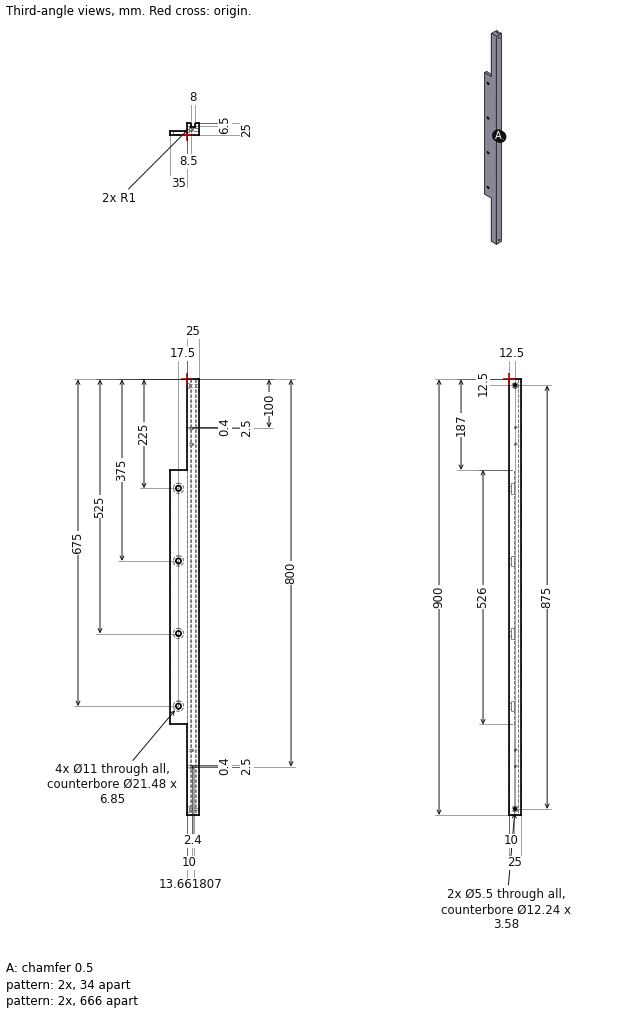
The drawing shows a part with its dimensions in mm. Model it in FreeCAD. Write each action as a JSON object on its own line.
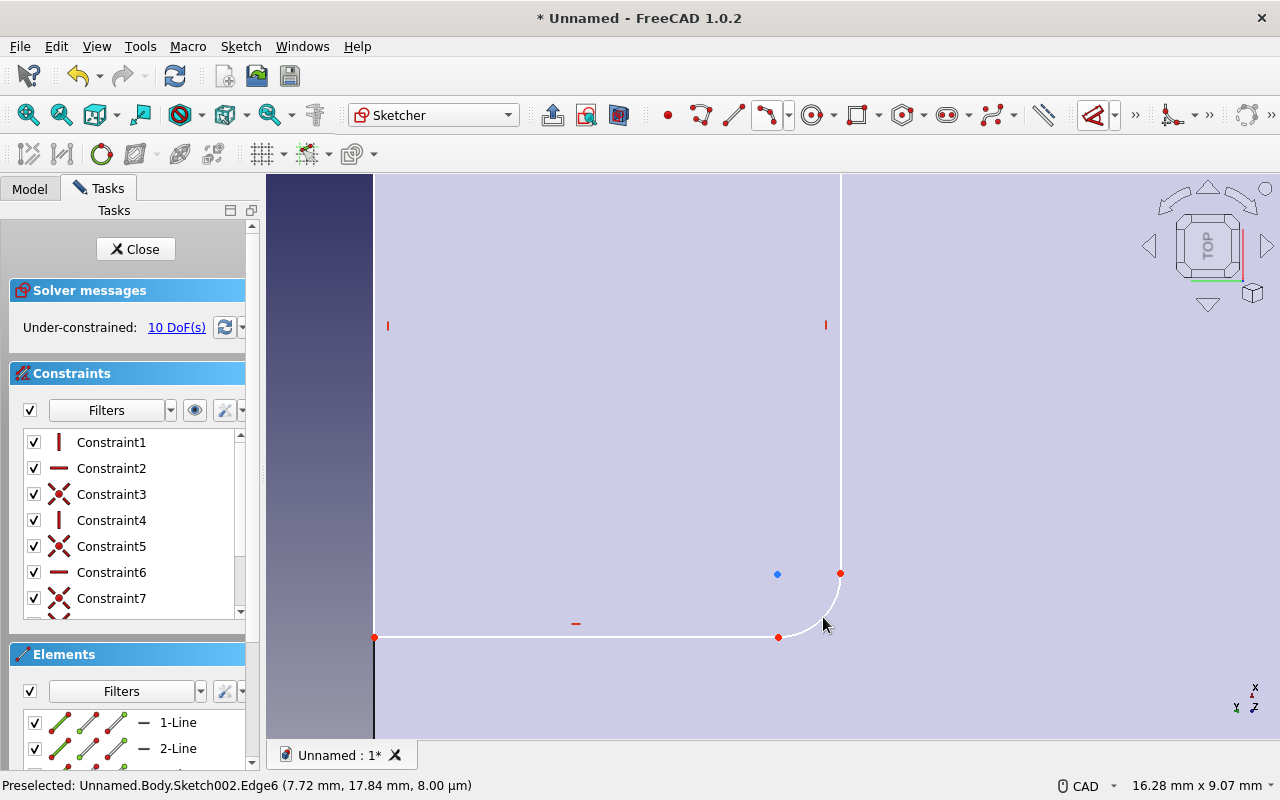
{"action": "left_click", "coordinate": [841, 424]}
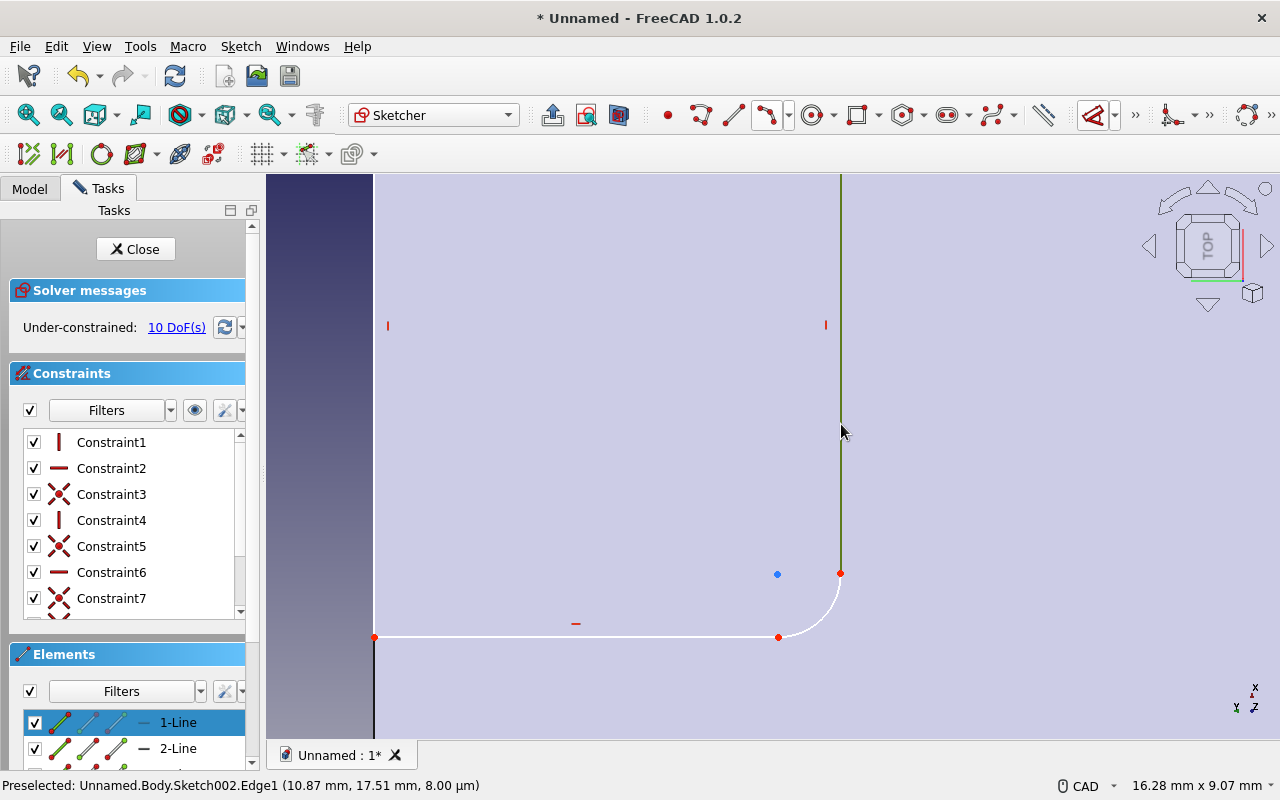
{"action": "scroll", "coordinate": [823, 618], "scroll_direction": "down", "scroll_amount": 3}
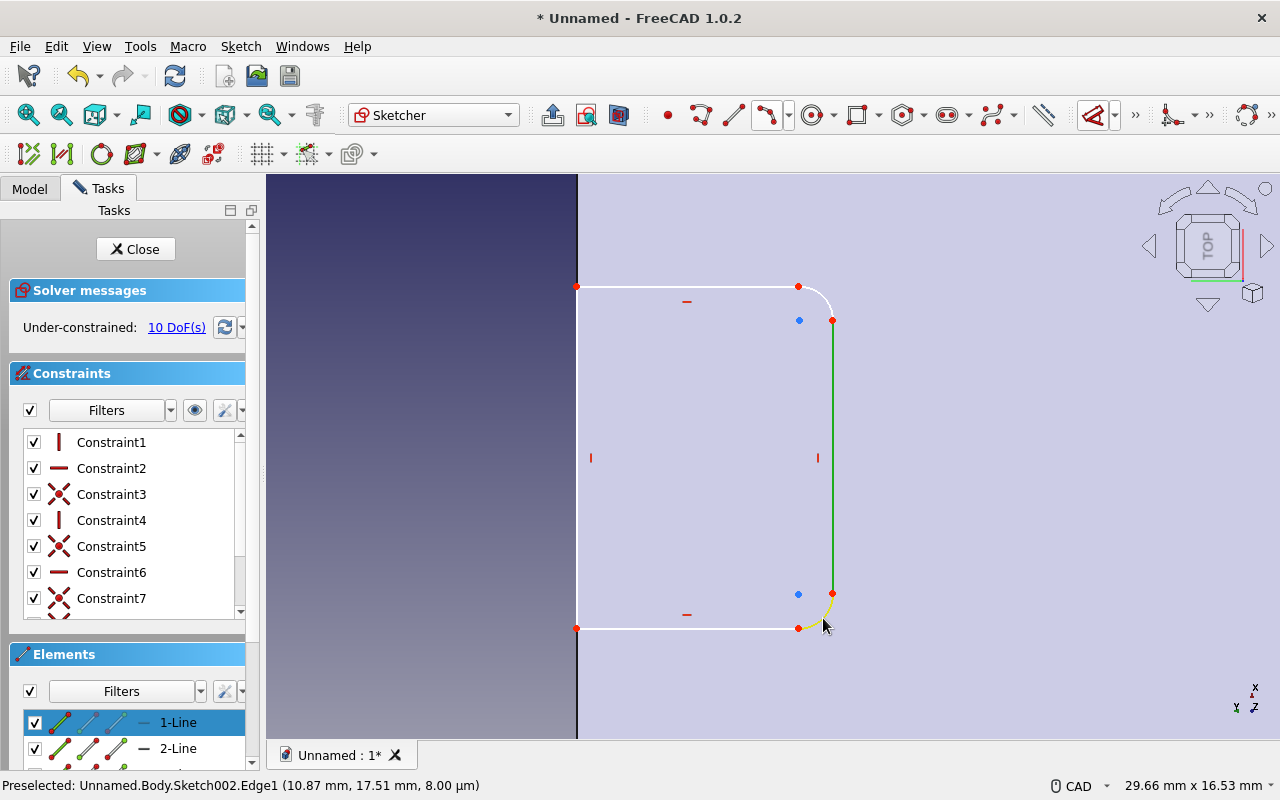
{"action": "left_click", "coordinate": [829, 305]}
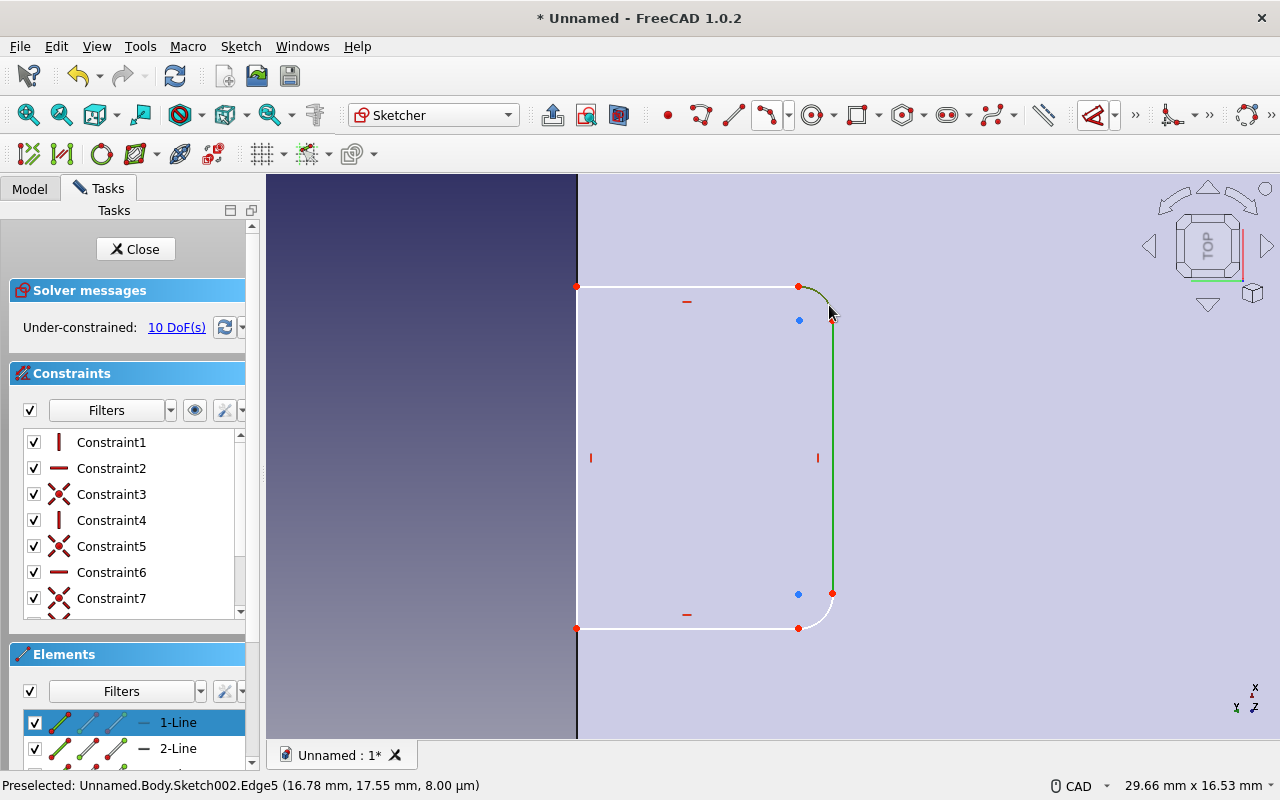
{"action": "key", "text": "t"}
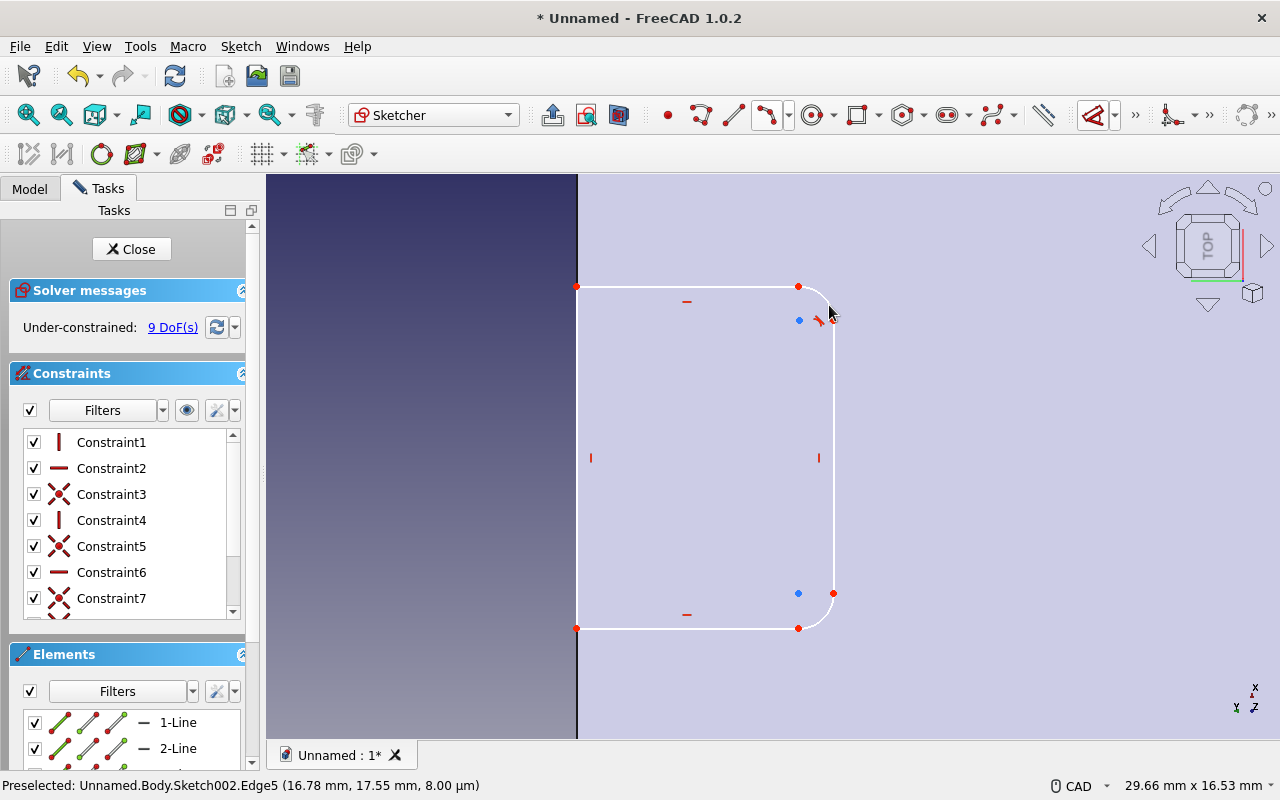
{"action": "left_click", "coordinate": [834, 512]}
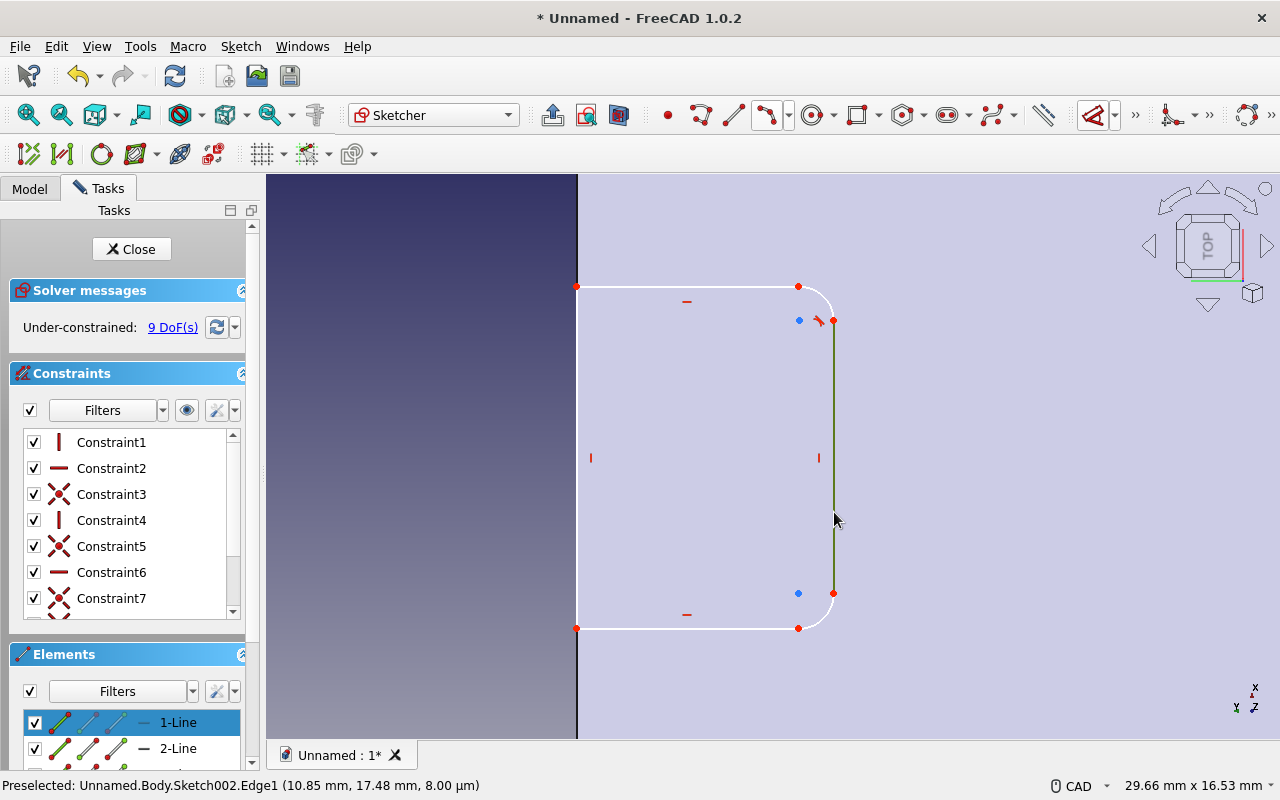
{"action": "left_click", "coordinate": [815, 625]}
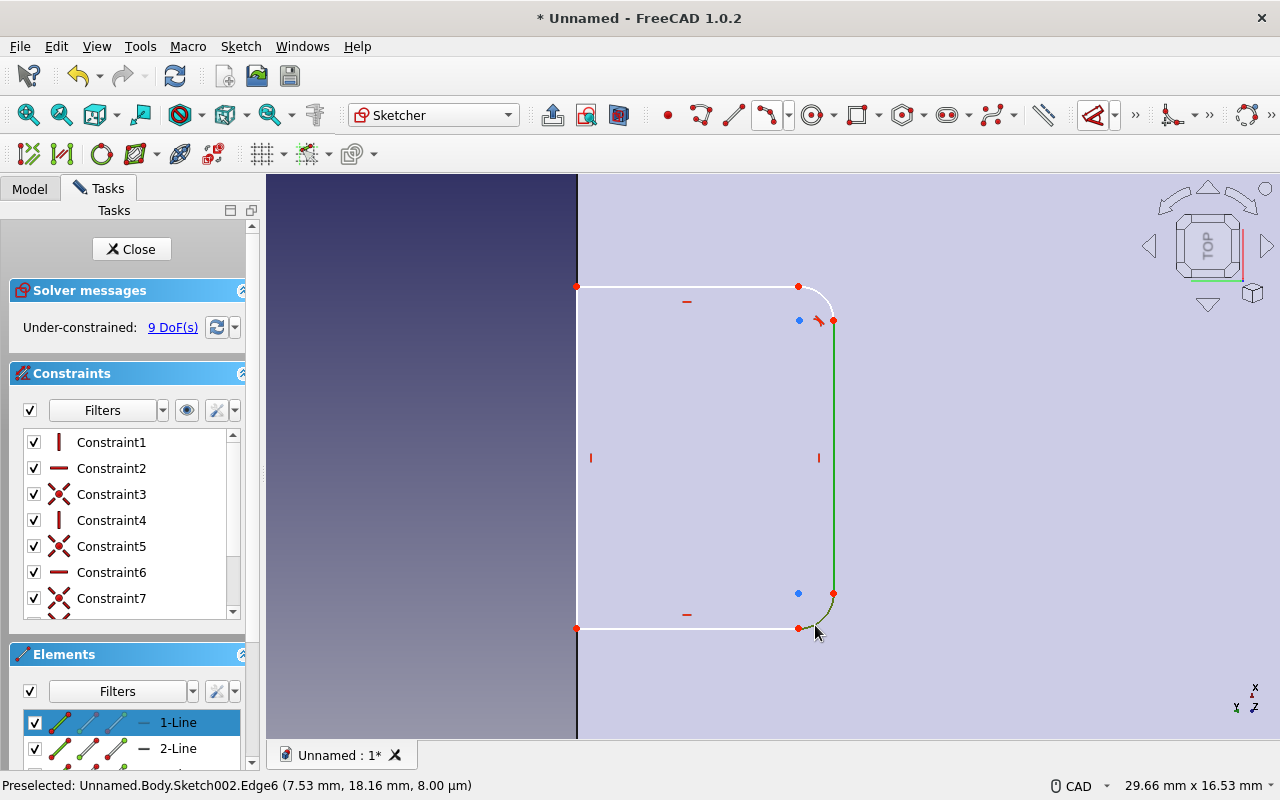
{"action": "key", "text": "t"}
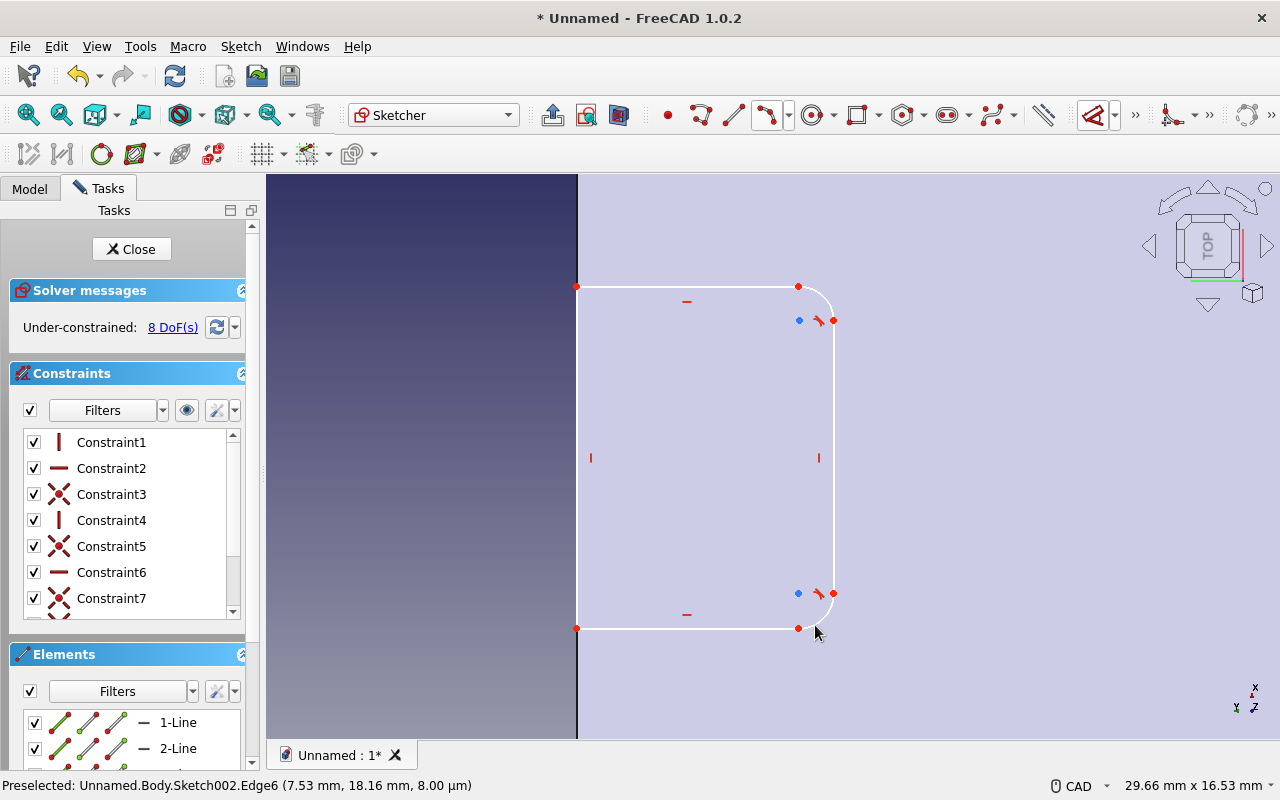
{"action": "left_click", "coordinate": [732, 287]}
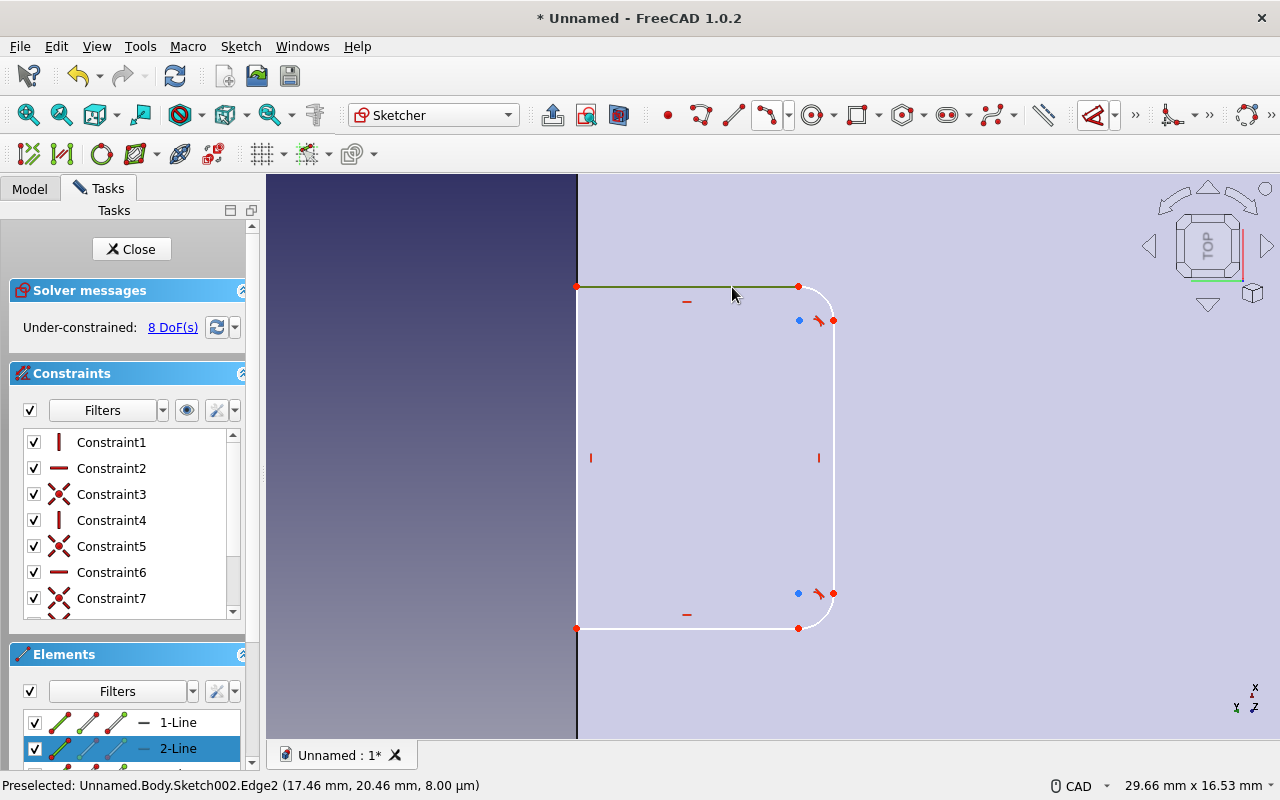
{"action": "left_click", "coordinate": [830, 305]}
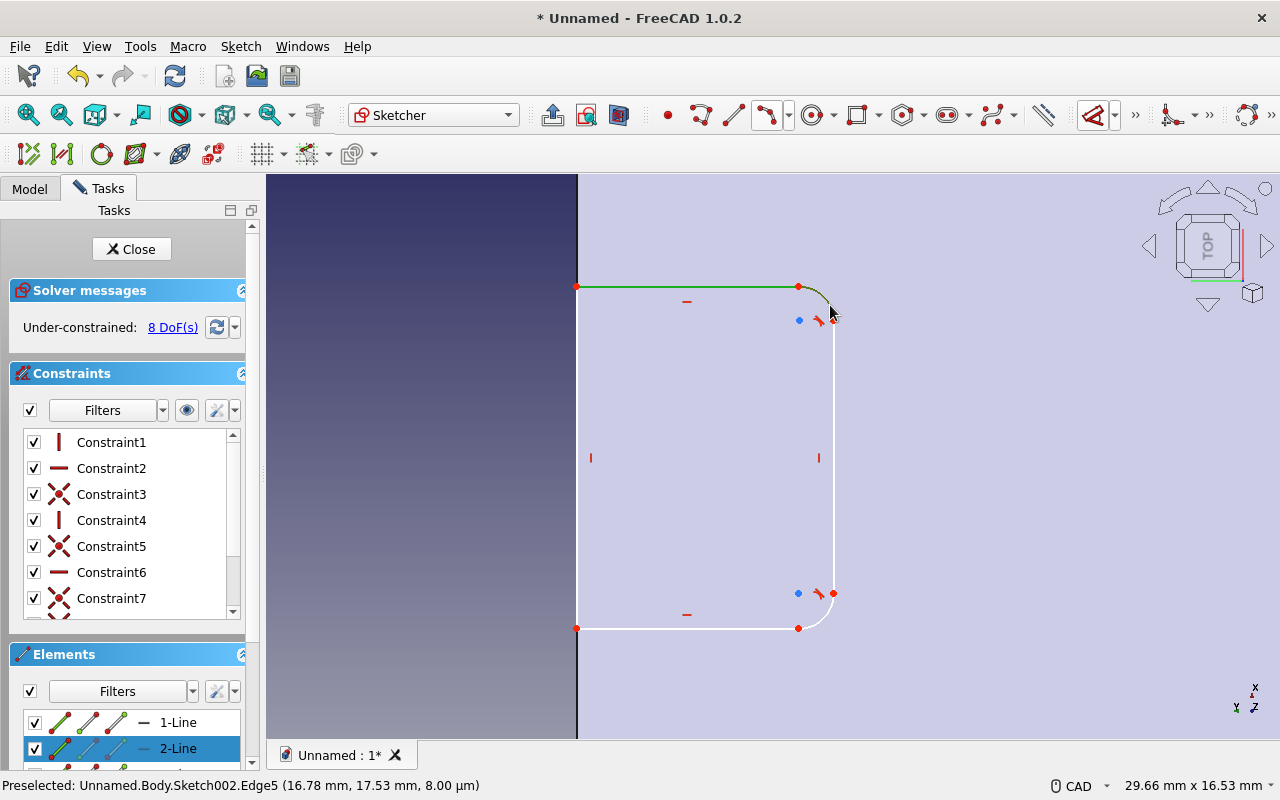
{"action": "key", "text": "t"}